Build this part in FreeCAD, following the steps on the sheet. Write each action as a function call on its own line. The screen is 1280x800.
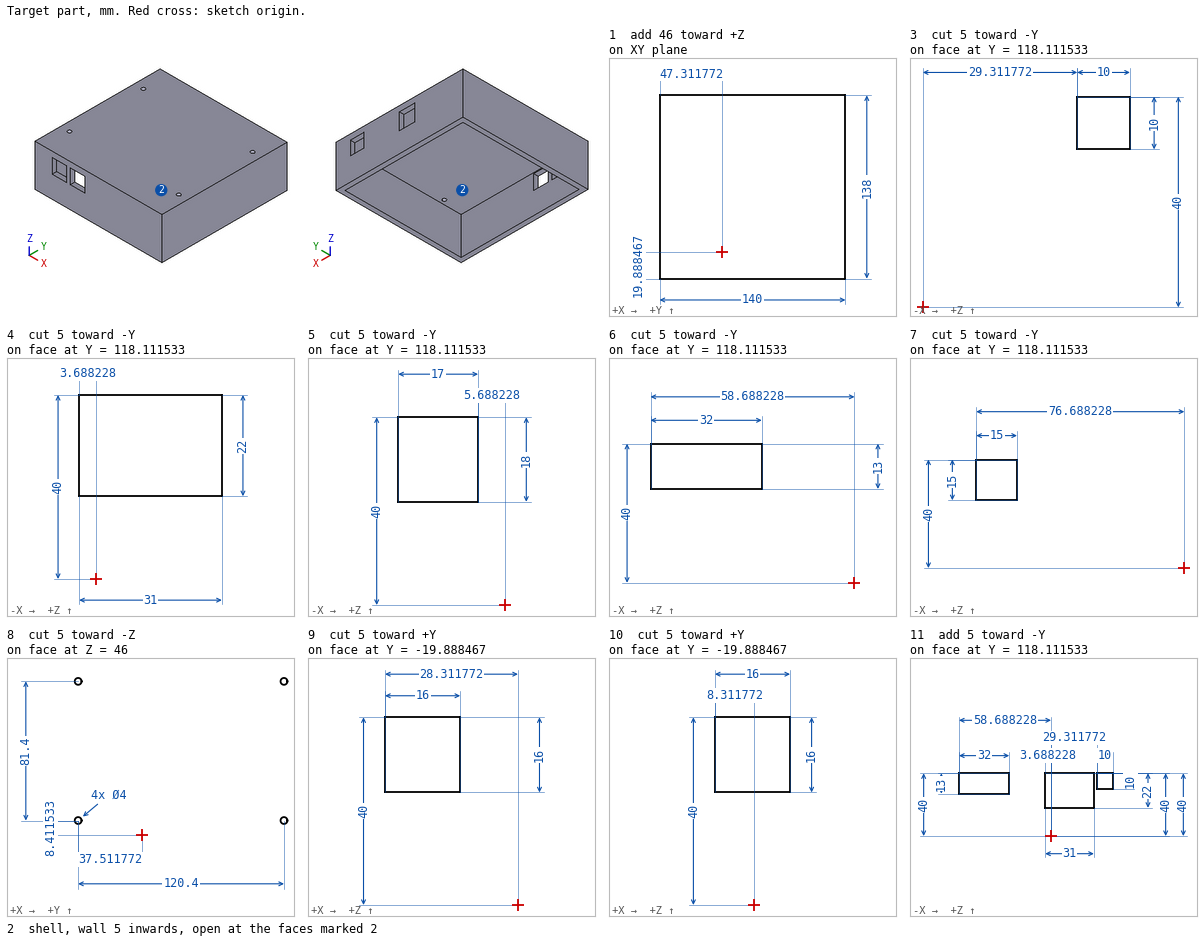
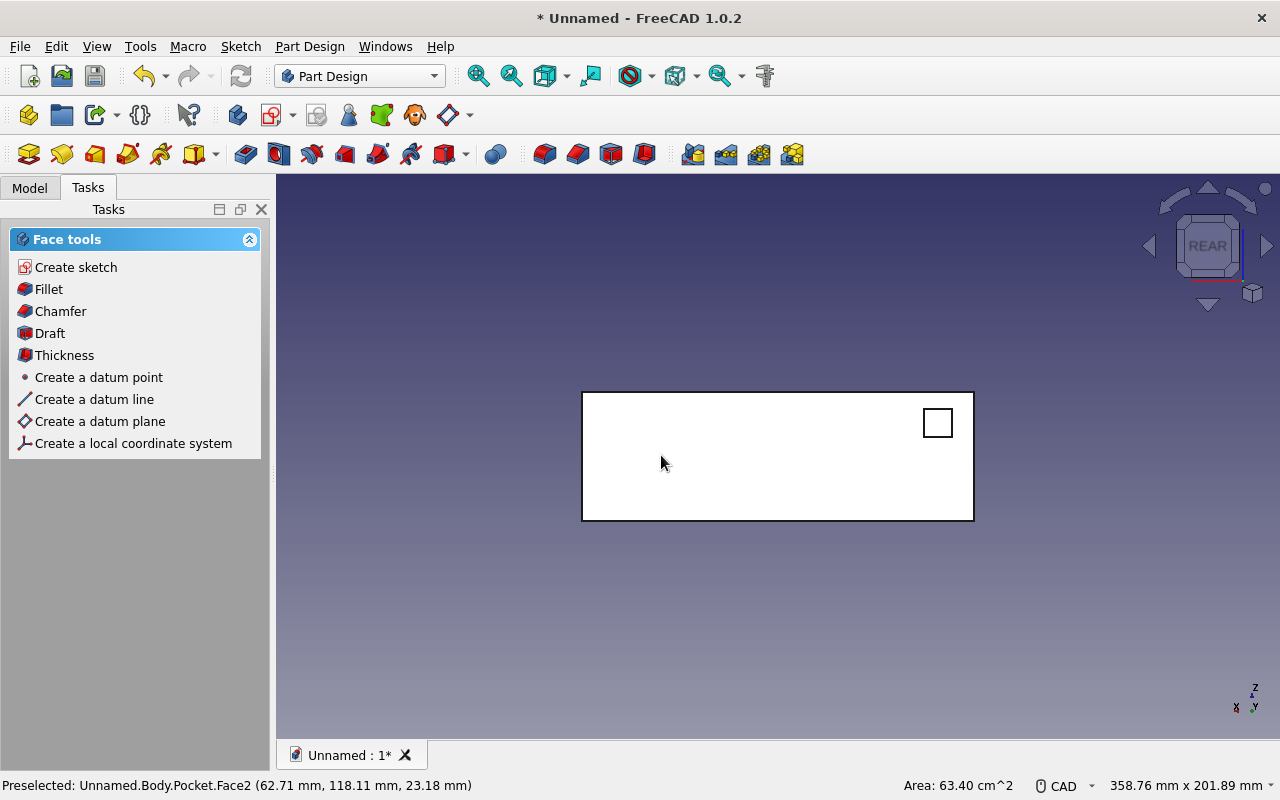
click(270, 116)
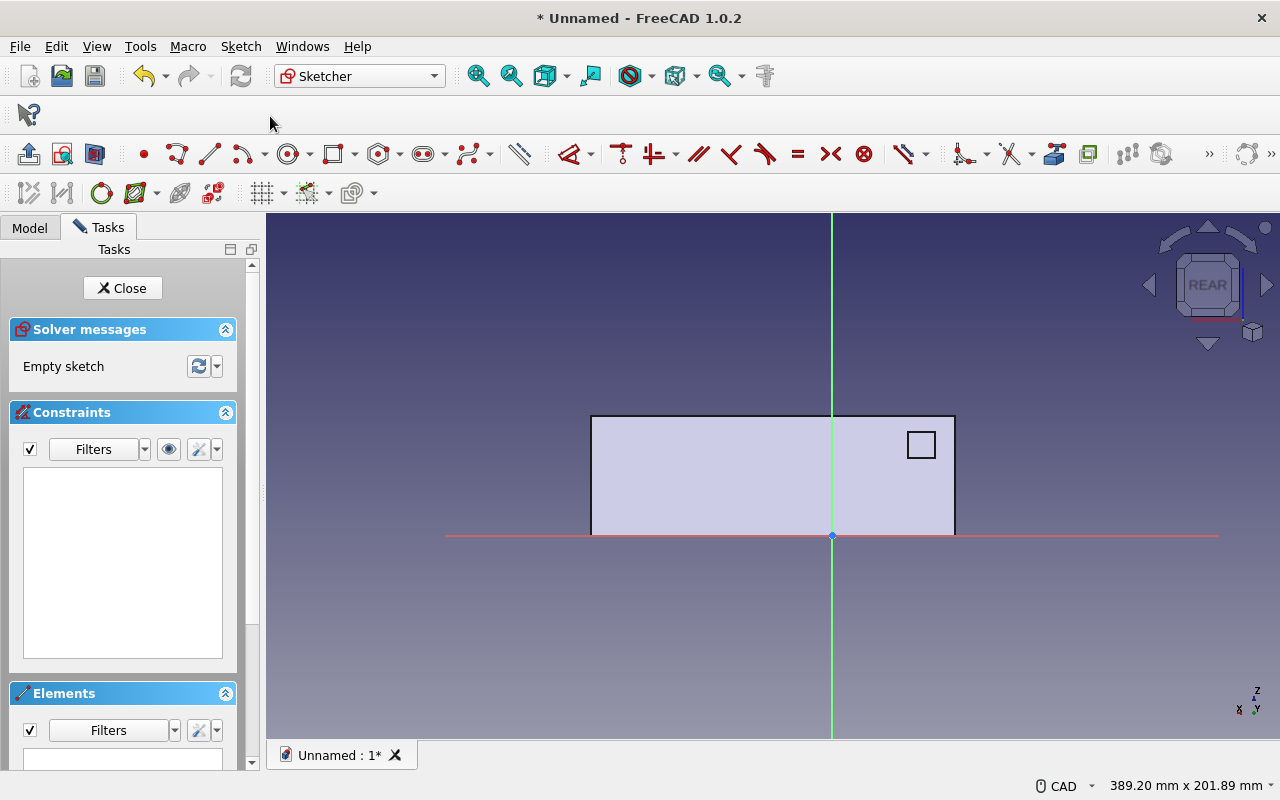
scroll(931, 487, up, 6)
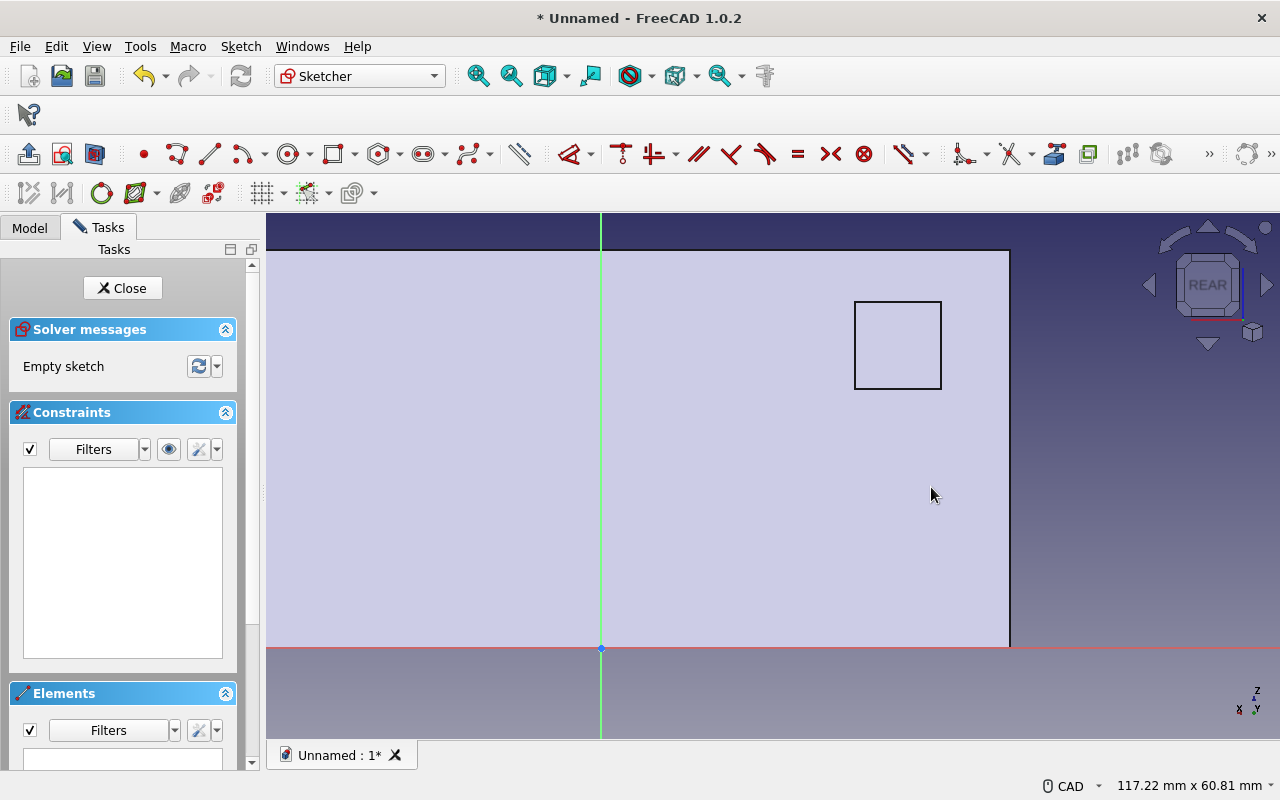
key(g)
key(r)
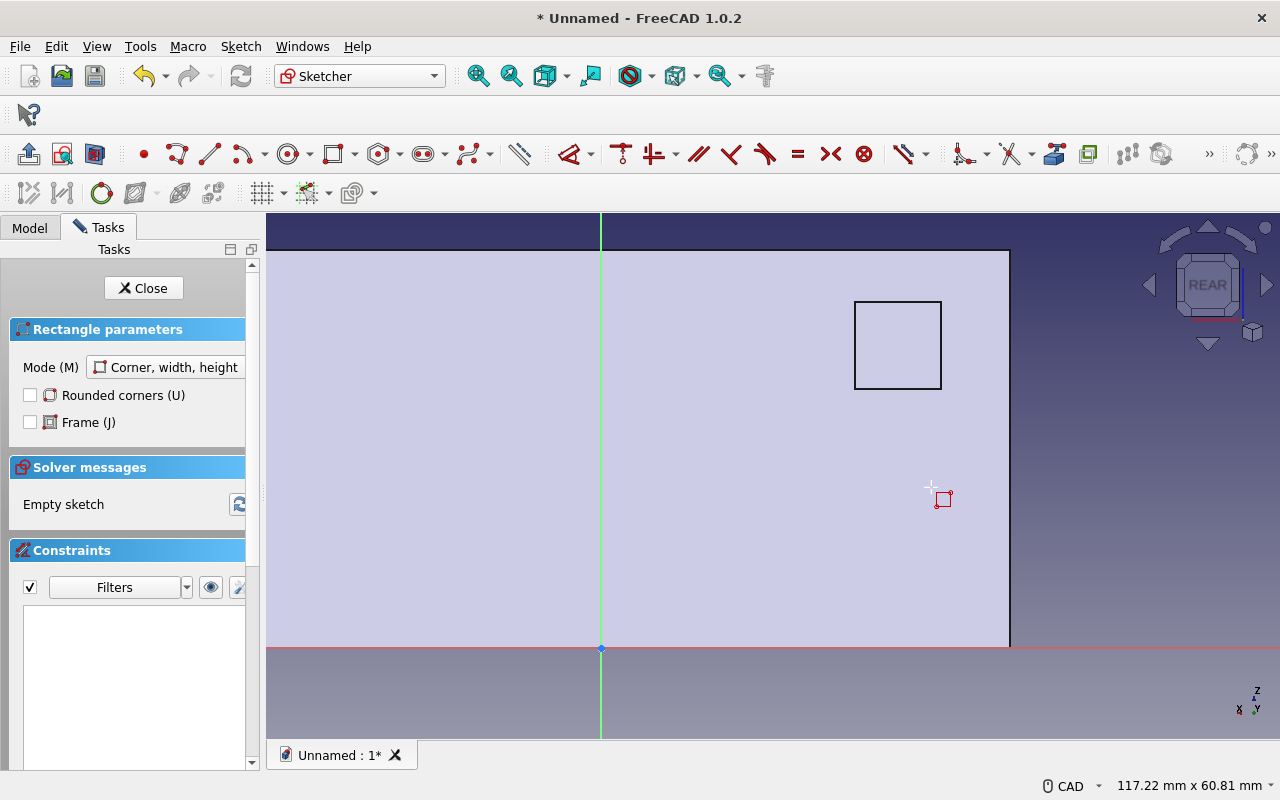
click(569, 302)
move(837, 493)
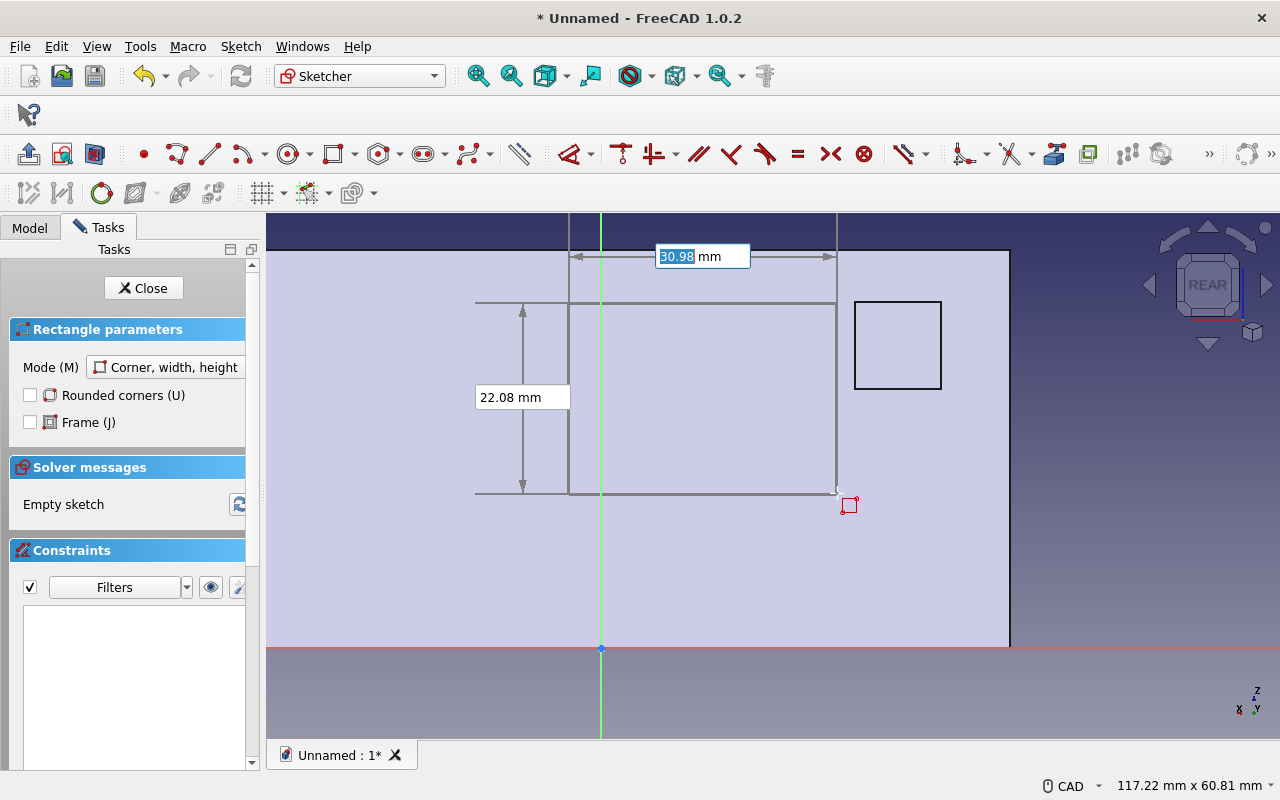
text(31)
key(Tab)
text(22)
key(Return)
key(Escape)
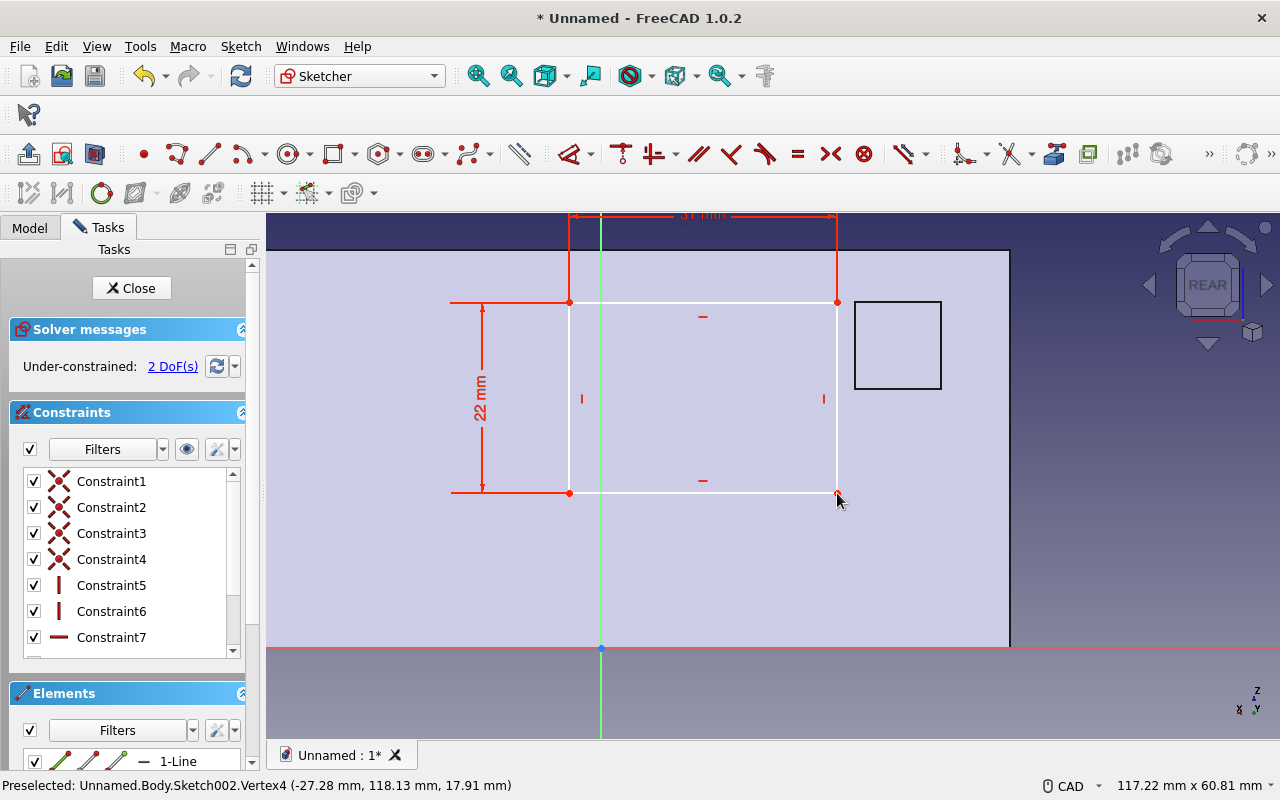
key(d)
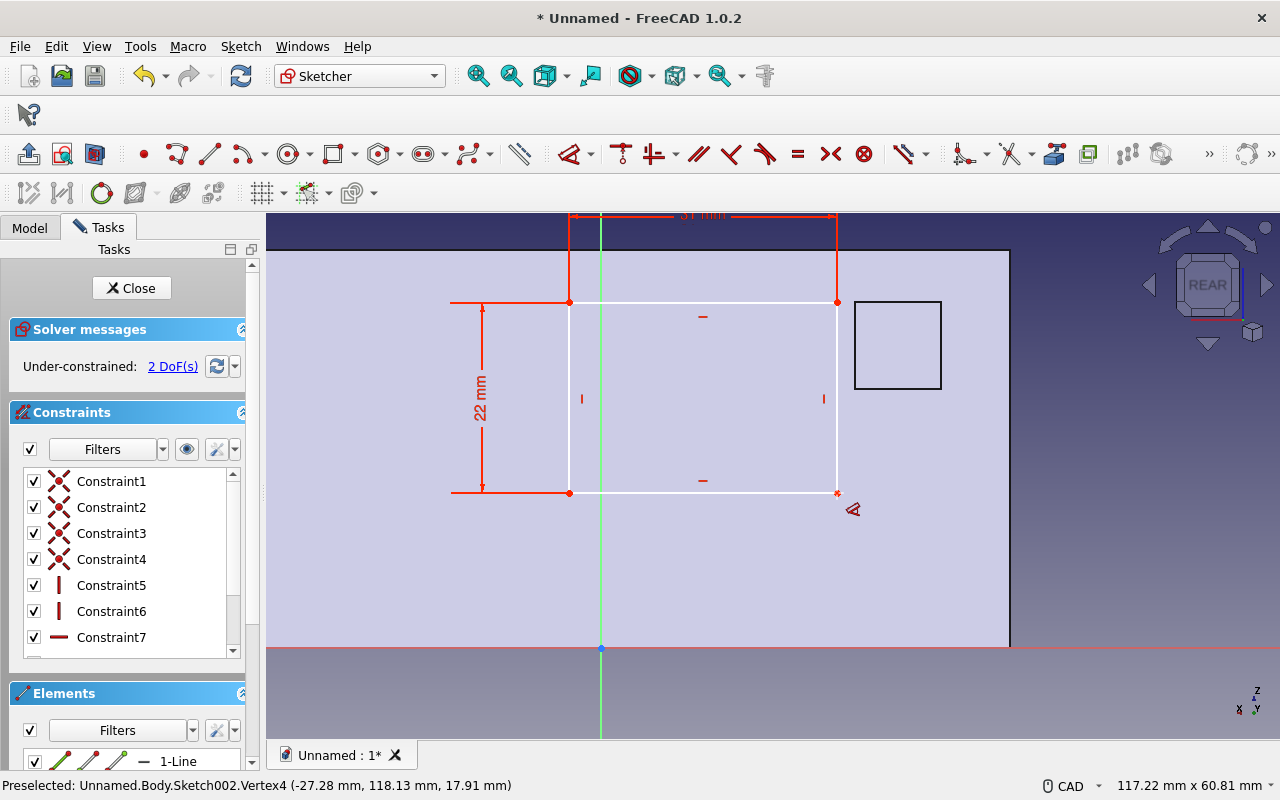
click(569, 303)
click(535, 476)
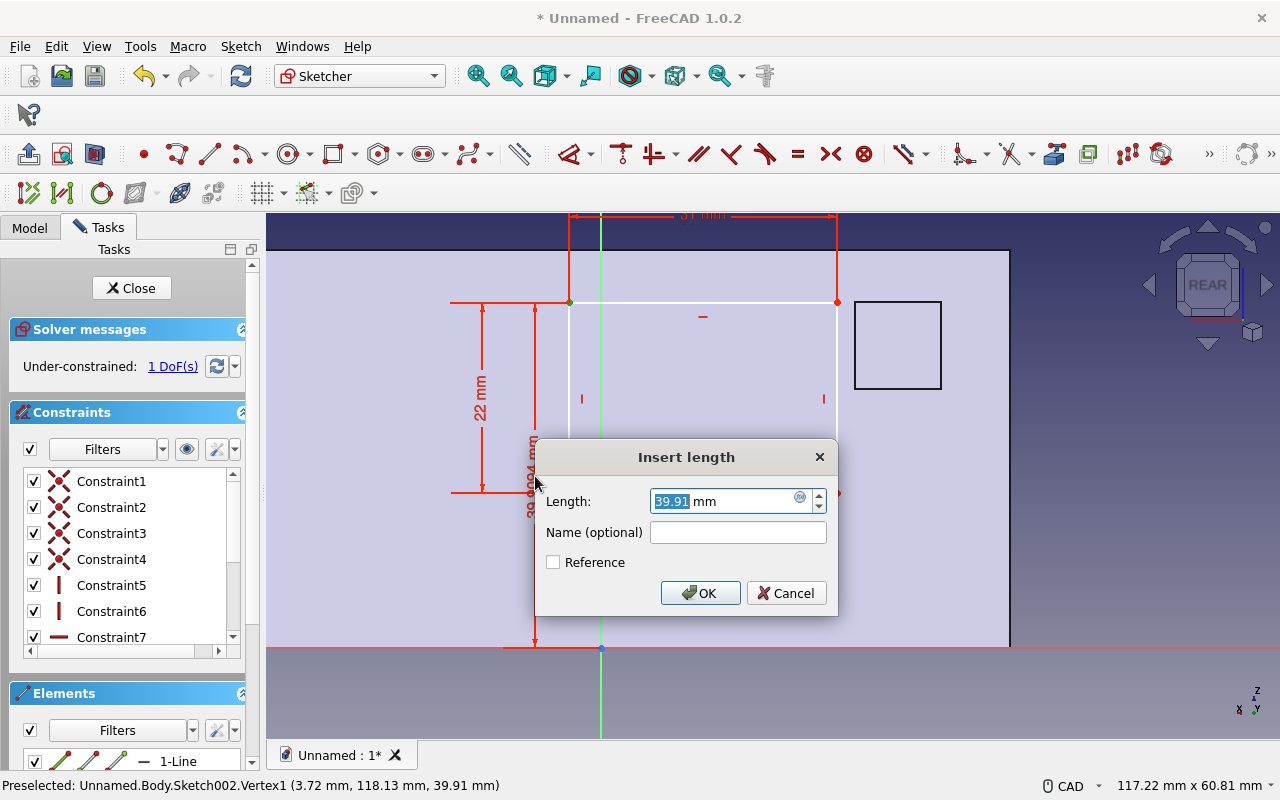
text(40)
key(Return)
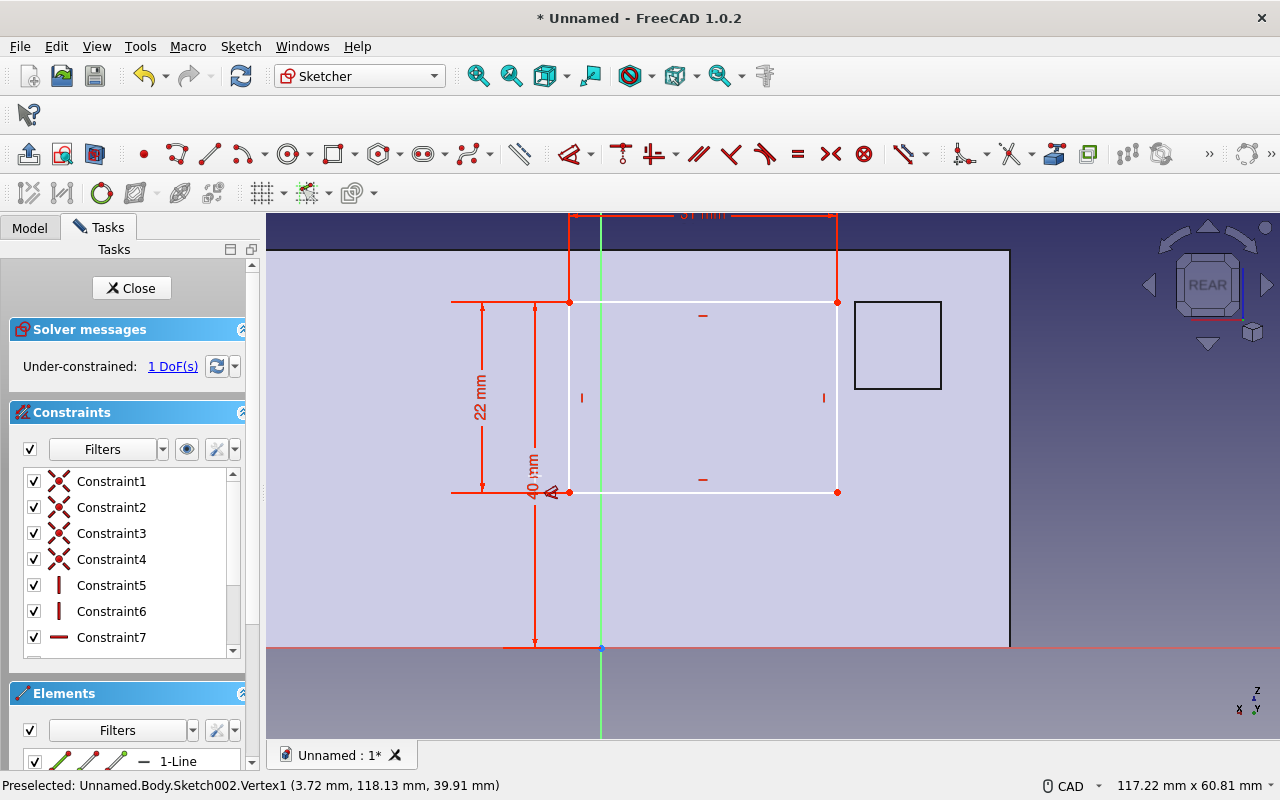
scroll(569, 302, up, 2)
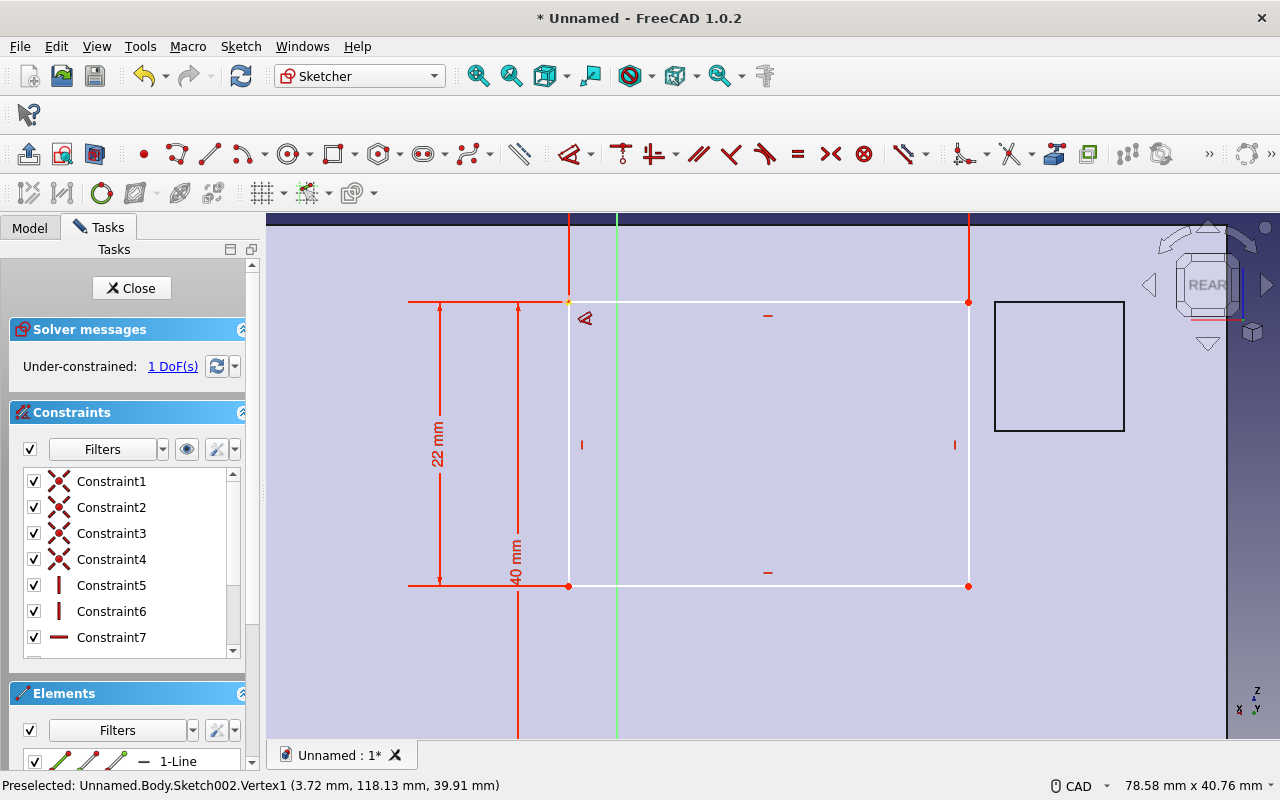
click(569, 302)
click(593, 268)